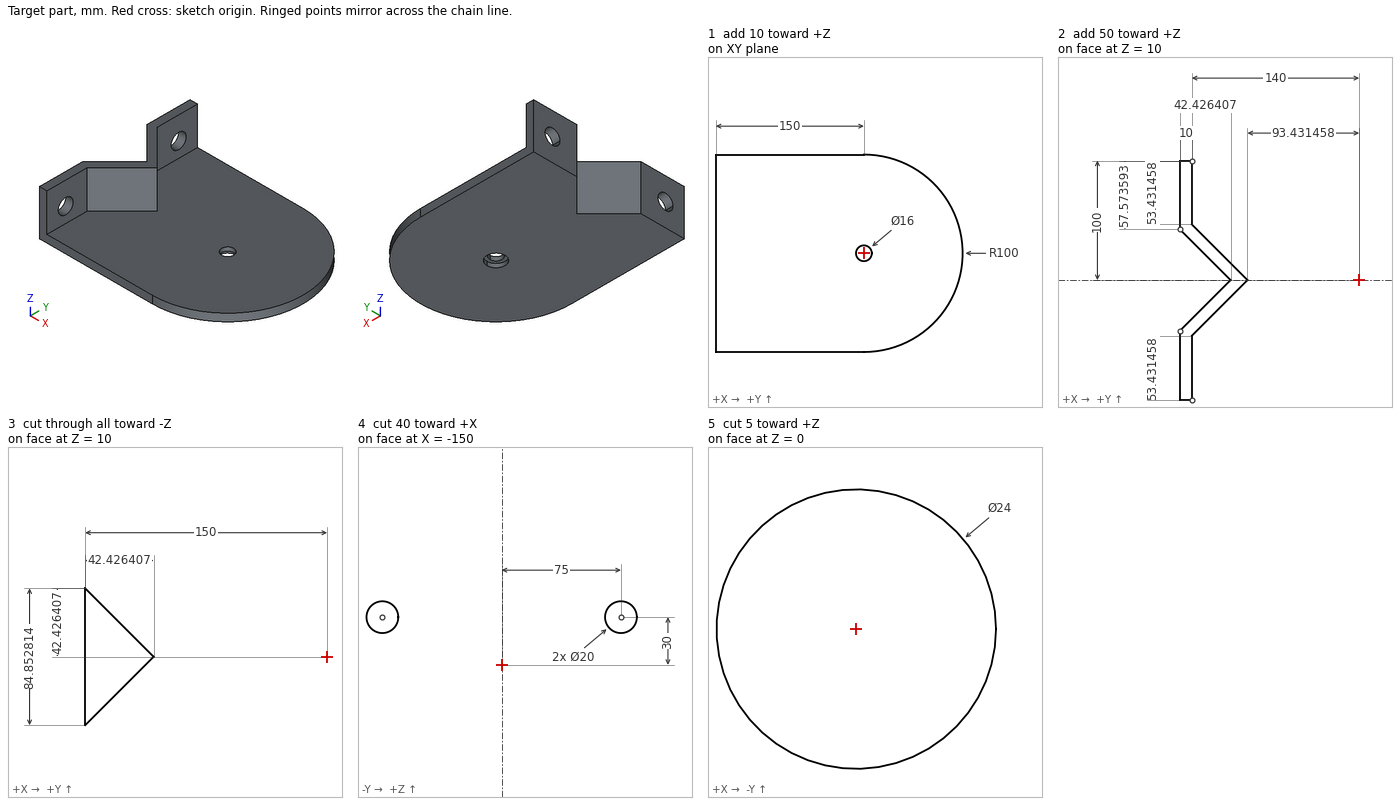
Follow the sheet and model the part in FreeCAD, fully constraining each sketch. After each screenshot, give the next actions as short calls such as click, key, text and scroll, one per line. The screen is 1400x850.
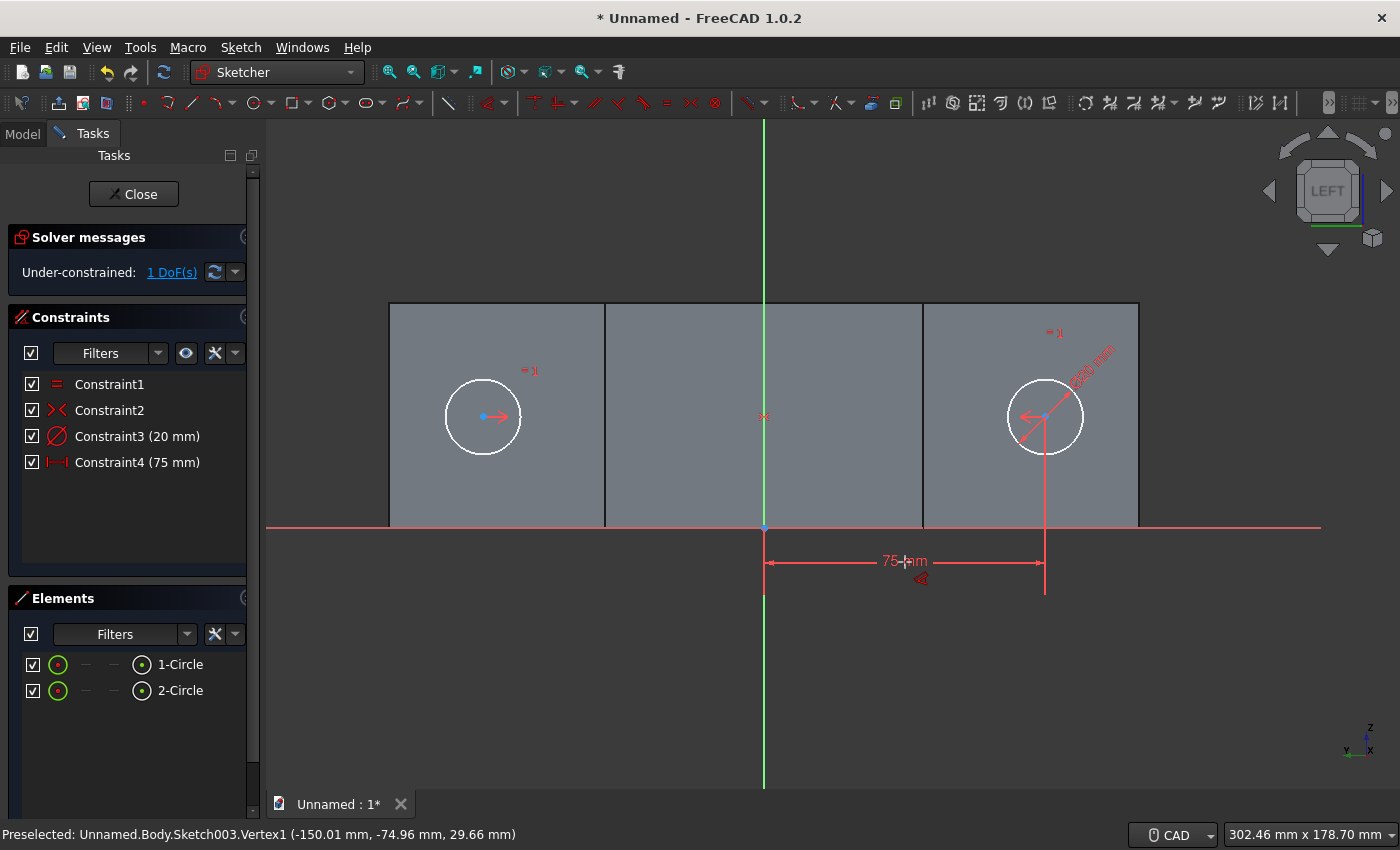
click(1045, 417)
click(1079, 473)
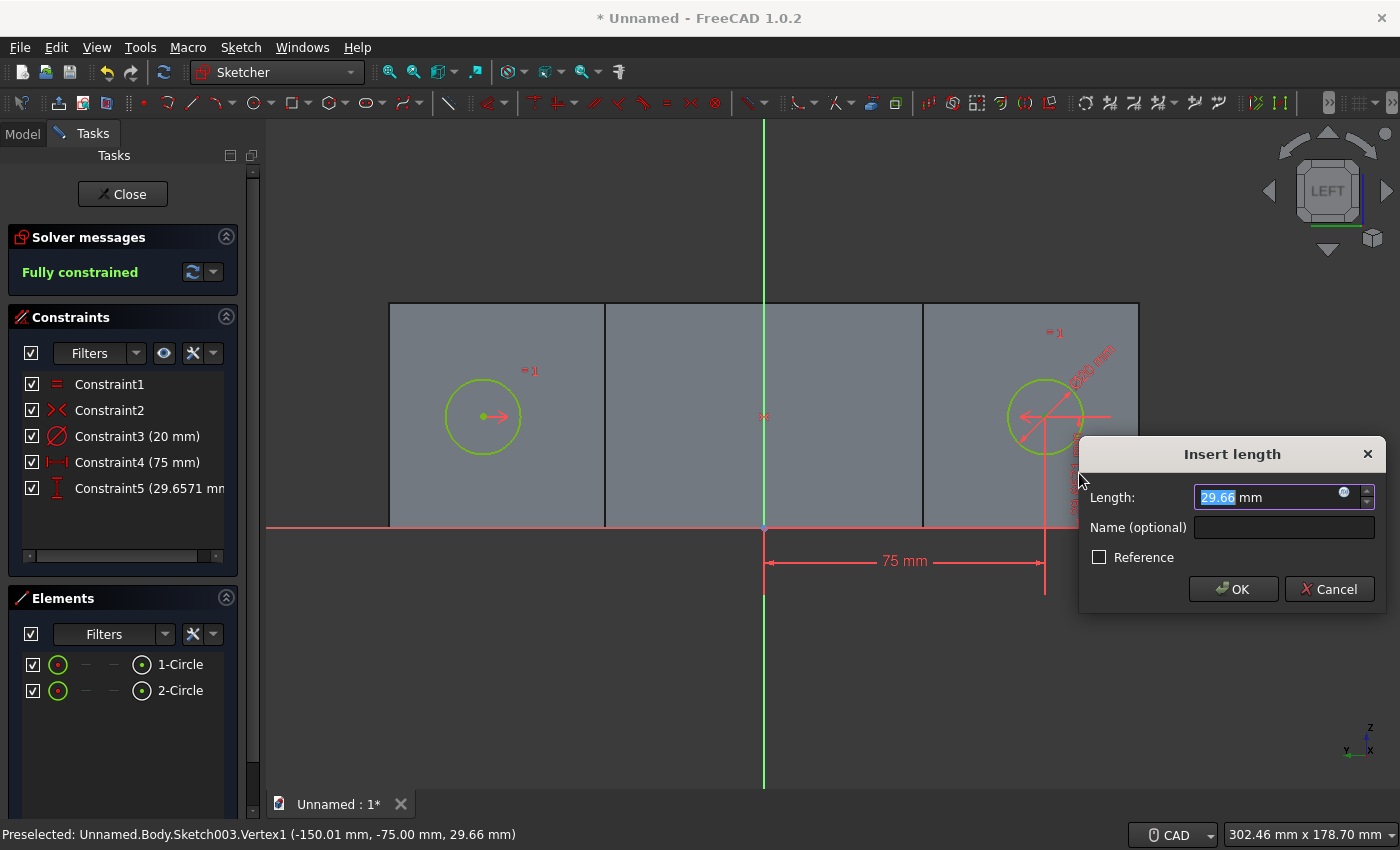
text(30)
key(Return)
key(Escape)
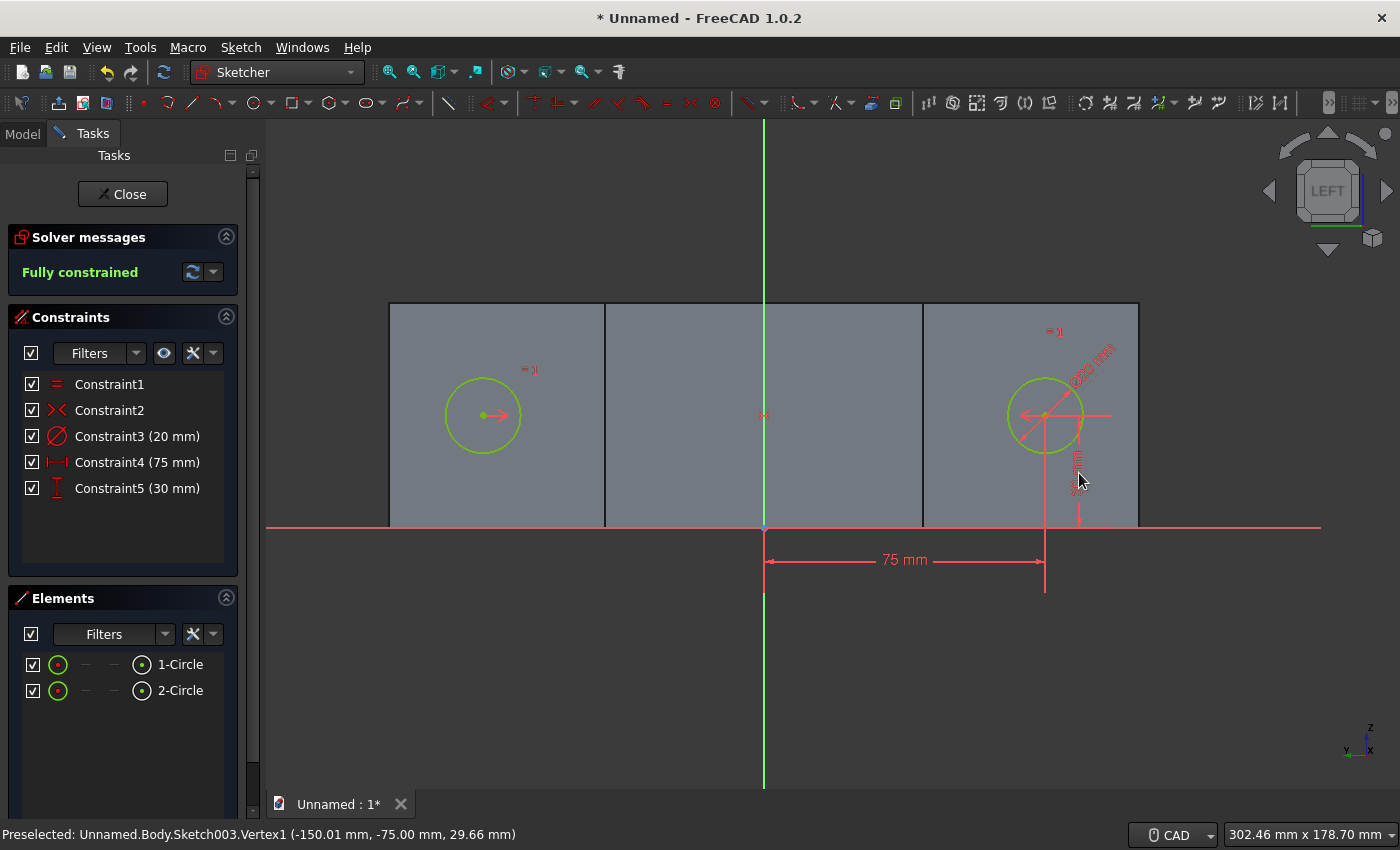
click(123, 194)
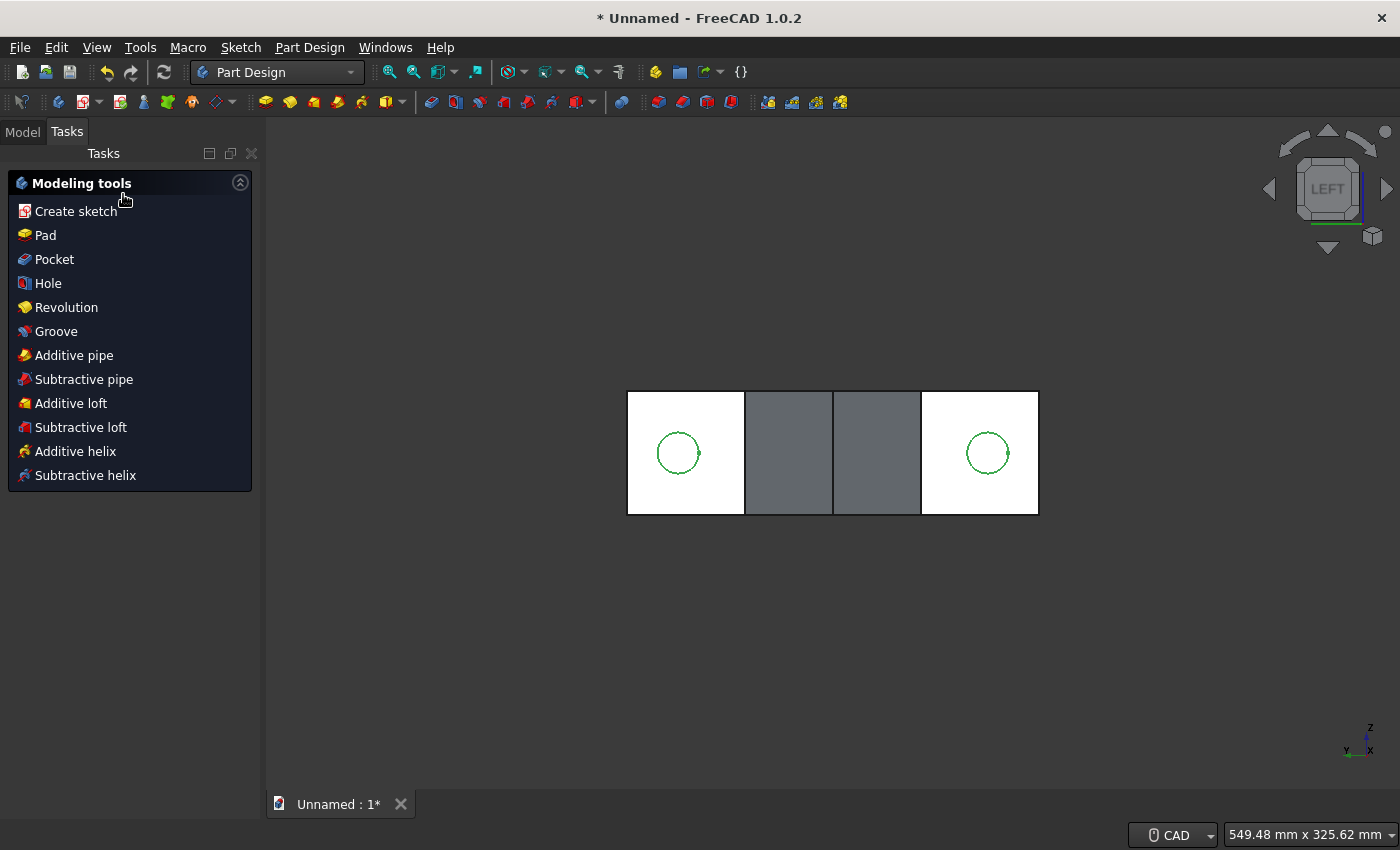
click(432, 102)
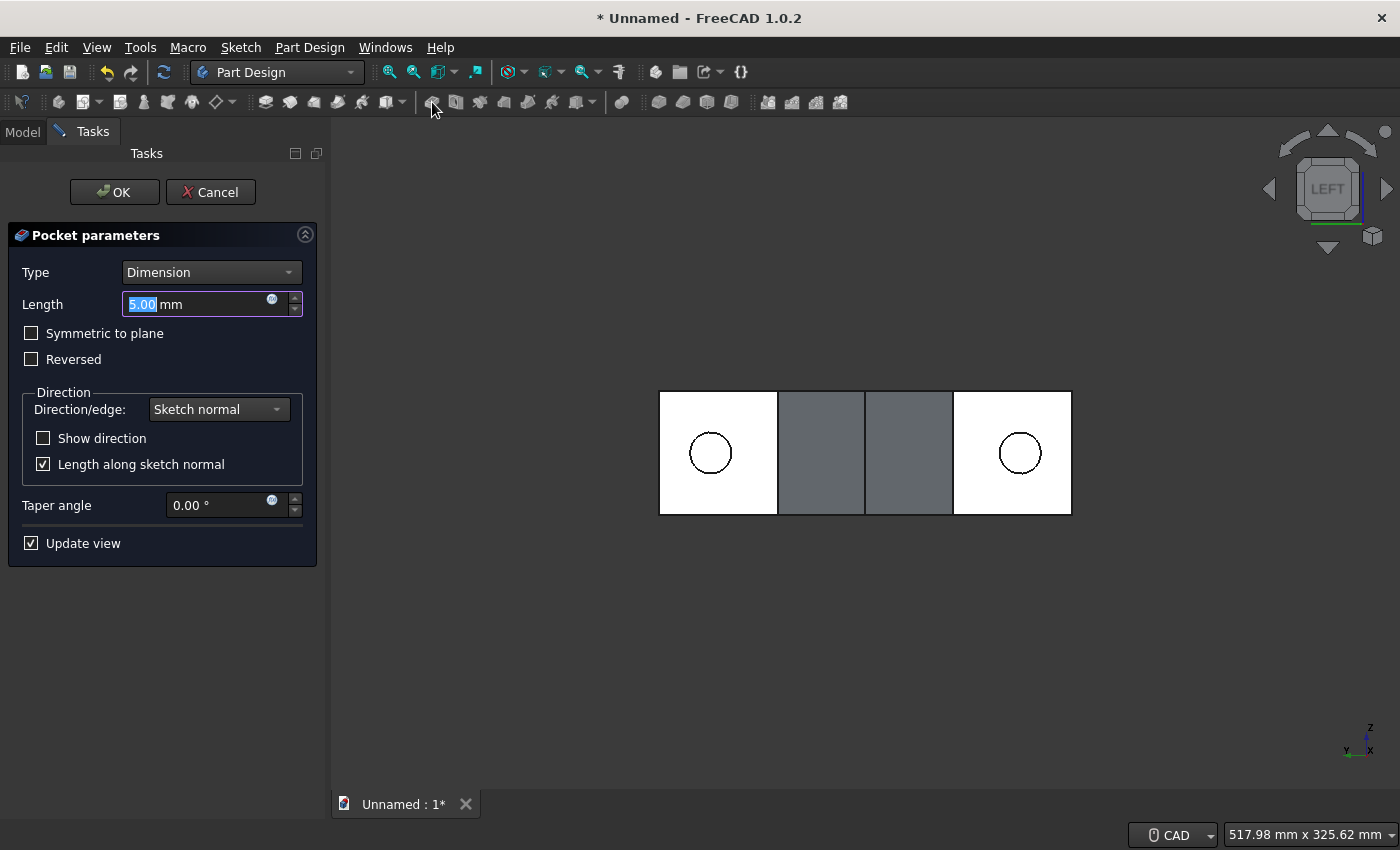
text(40)
key(Tab)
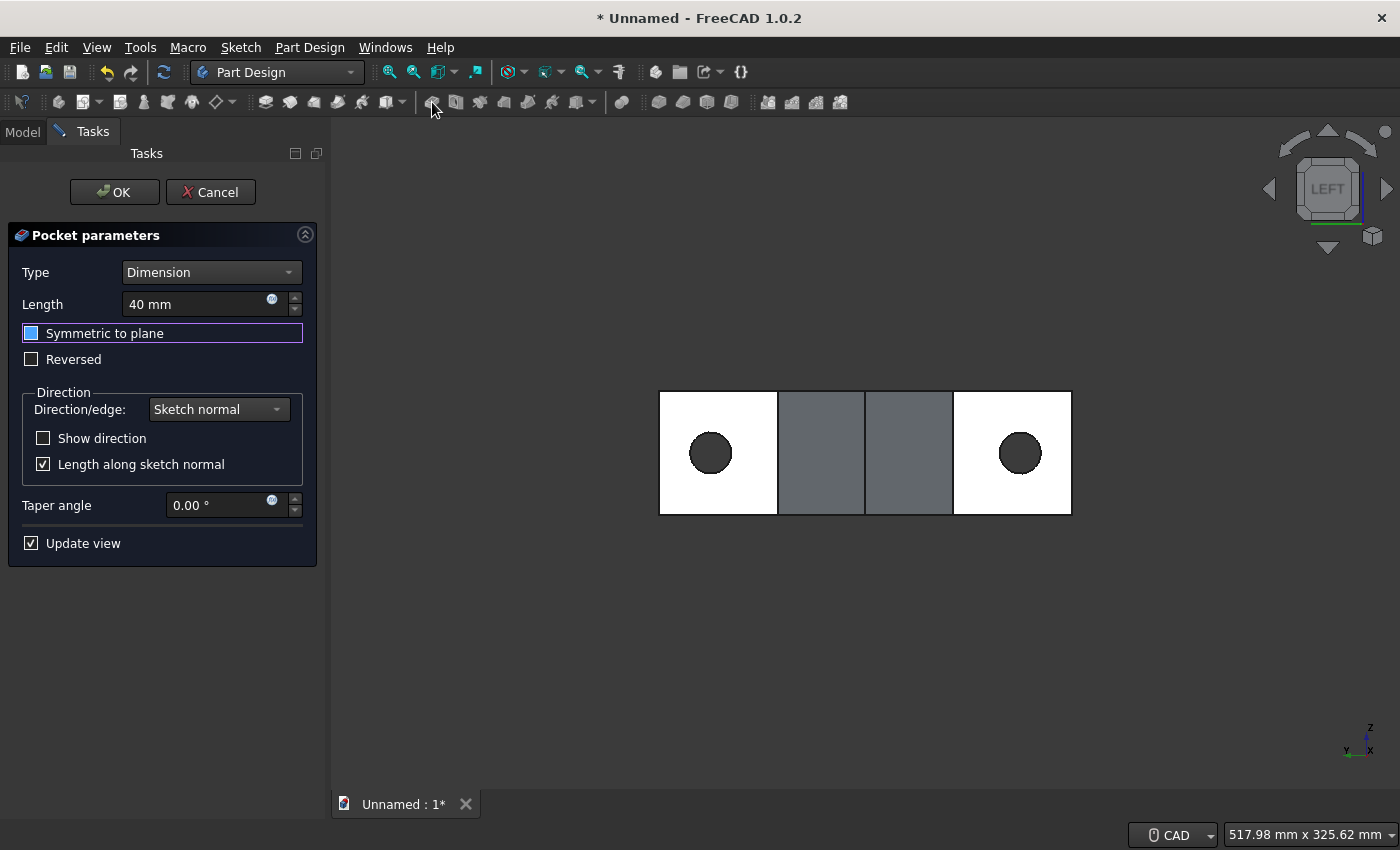
click(115, 192)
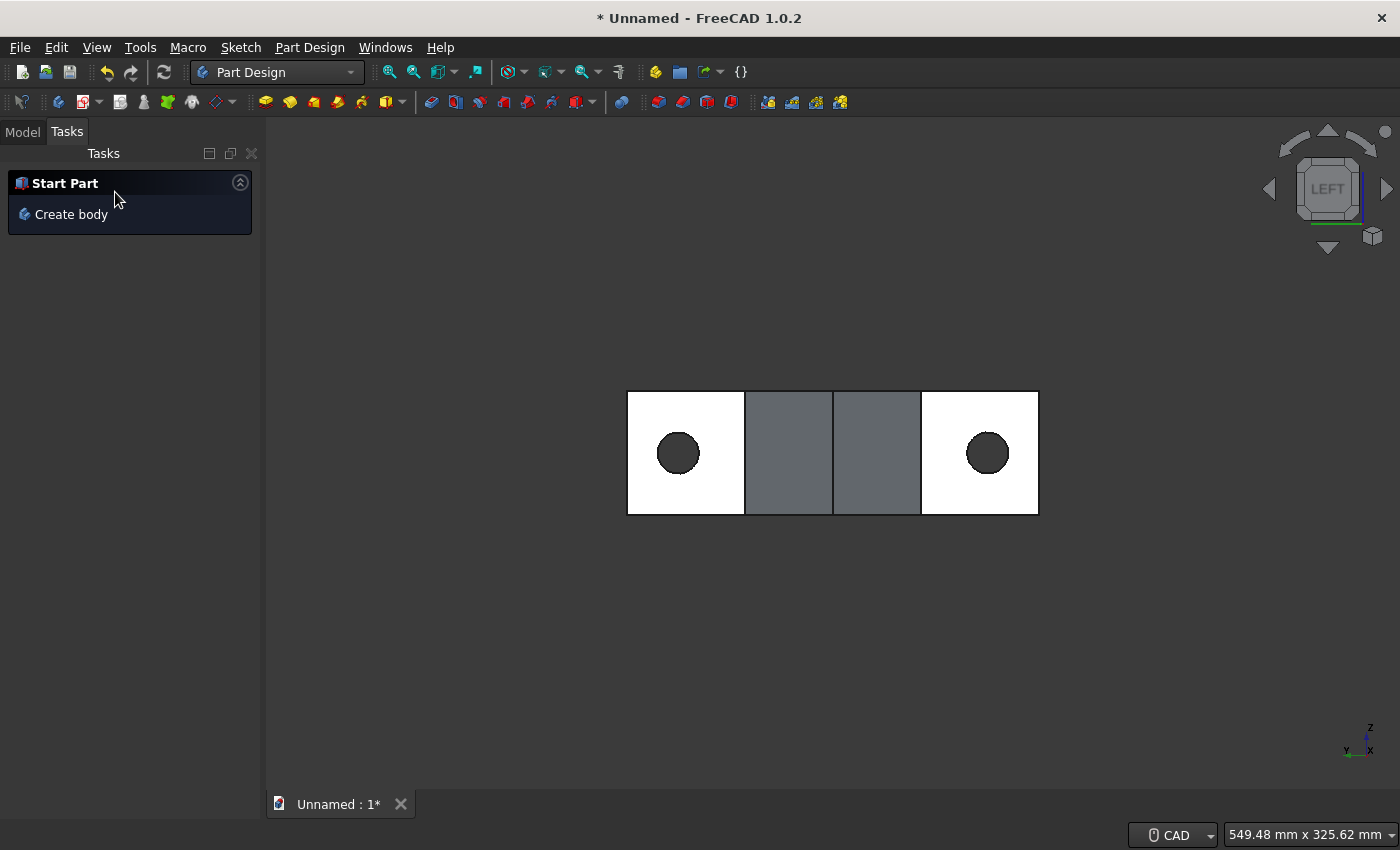
click(390, 72)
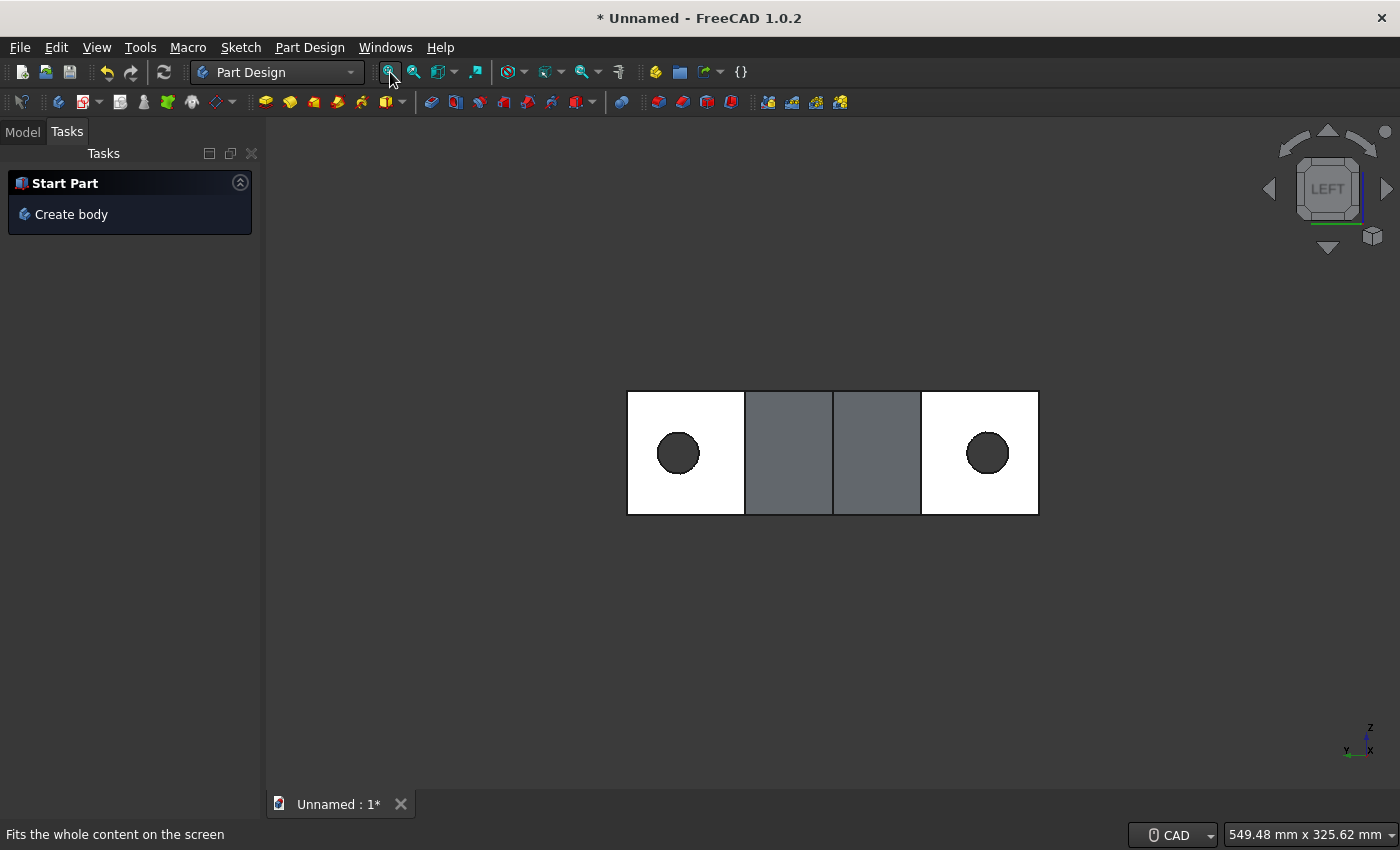
key(5)